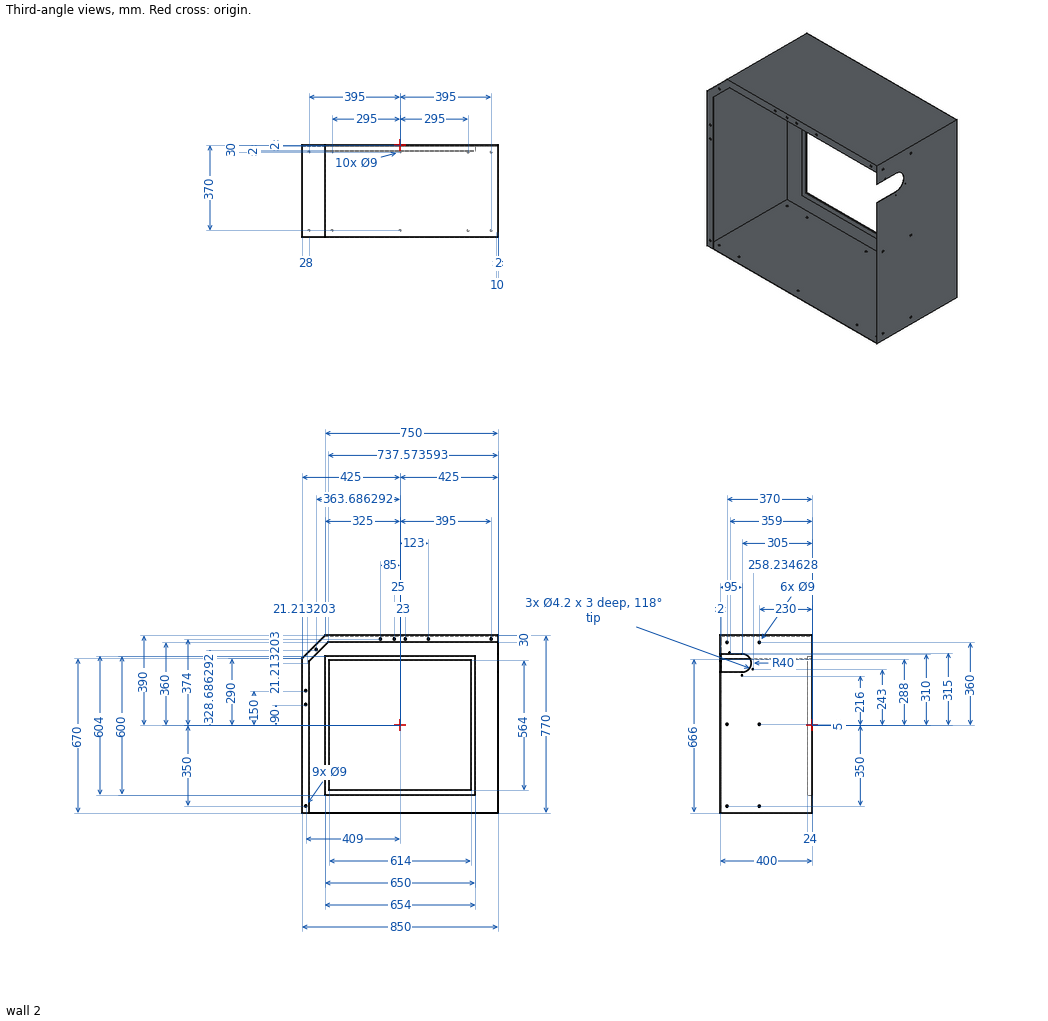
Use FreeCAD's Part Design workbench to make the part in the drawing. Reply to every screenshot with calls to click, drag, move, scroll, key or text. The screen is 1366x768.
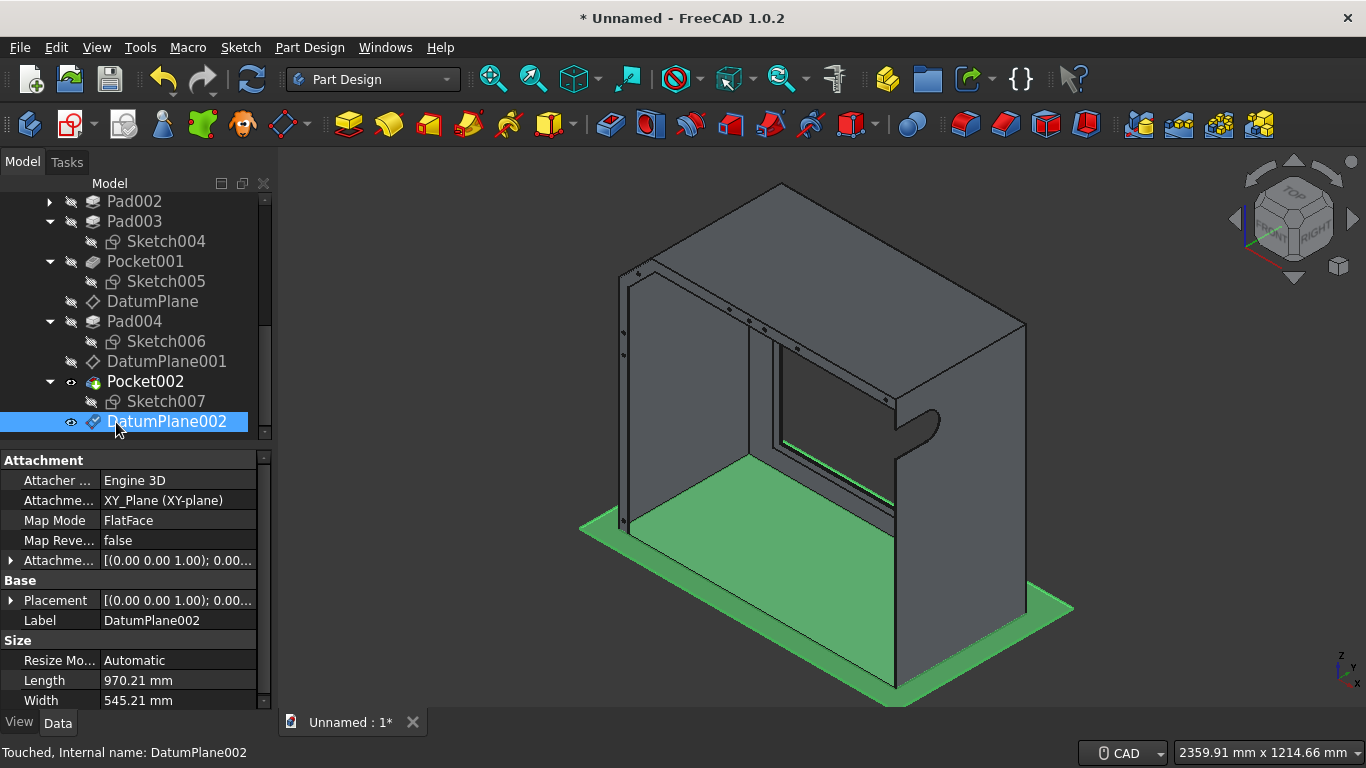
click(70, 124)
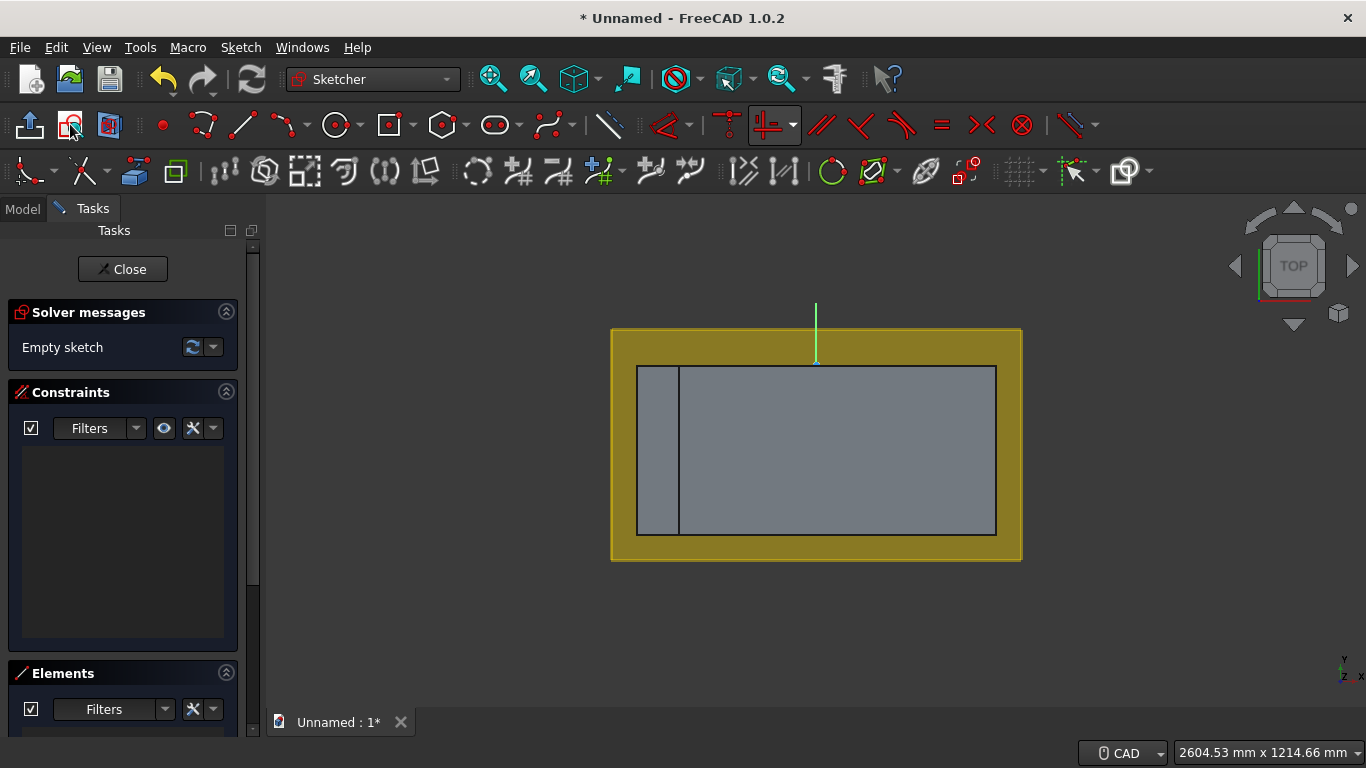
click(110, 126)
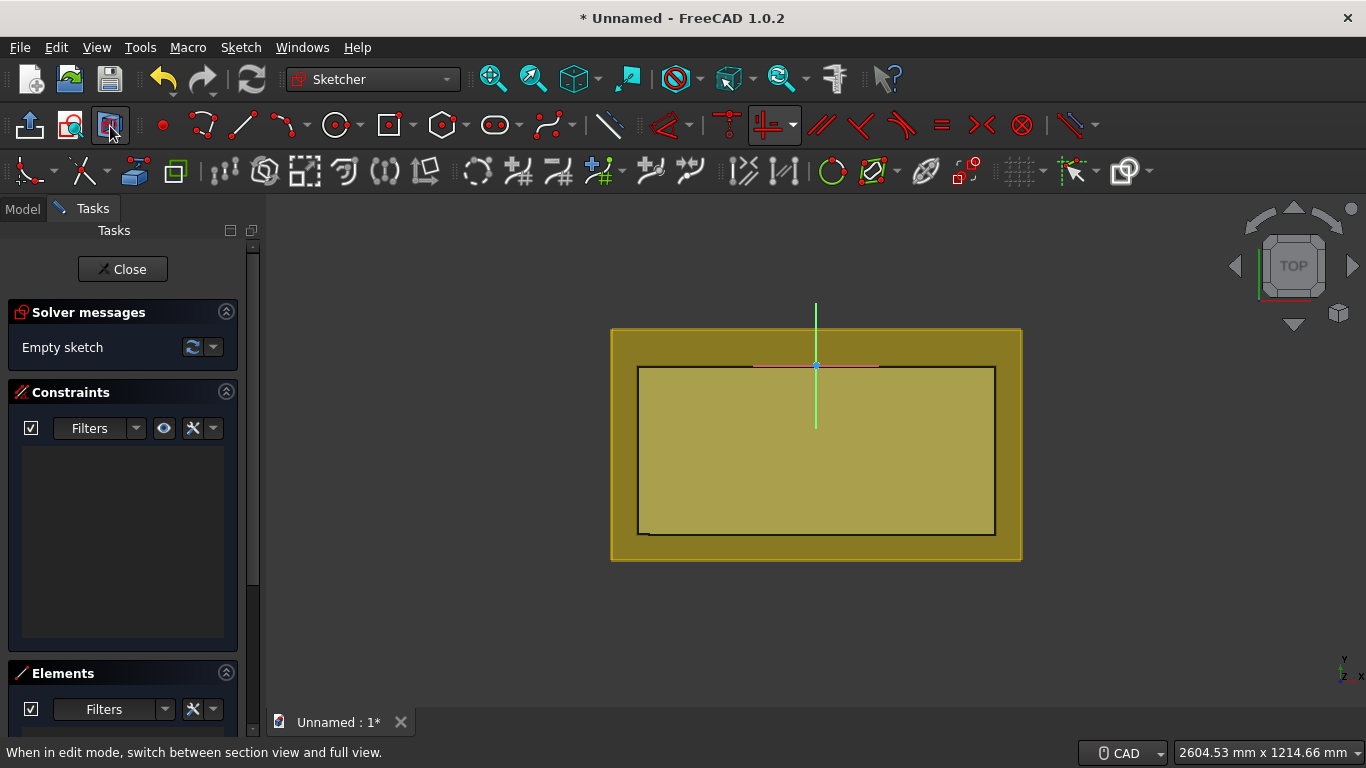
scroll(900, 438, up, 3)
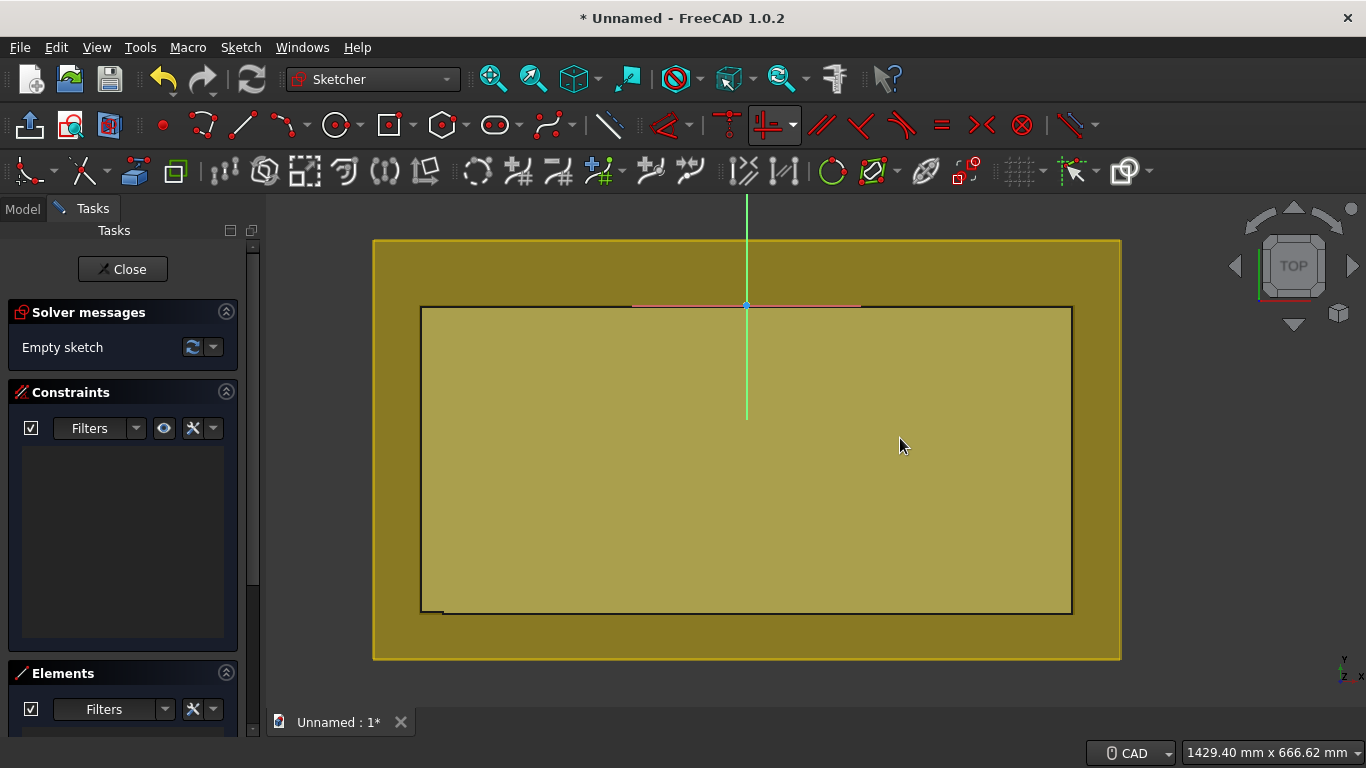
click(336, 126)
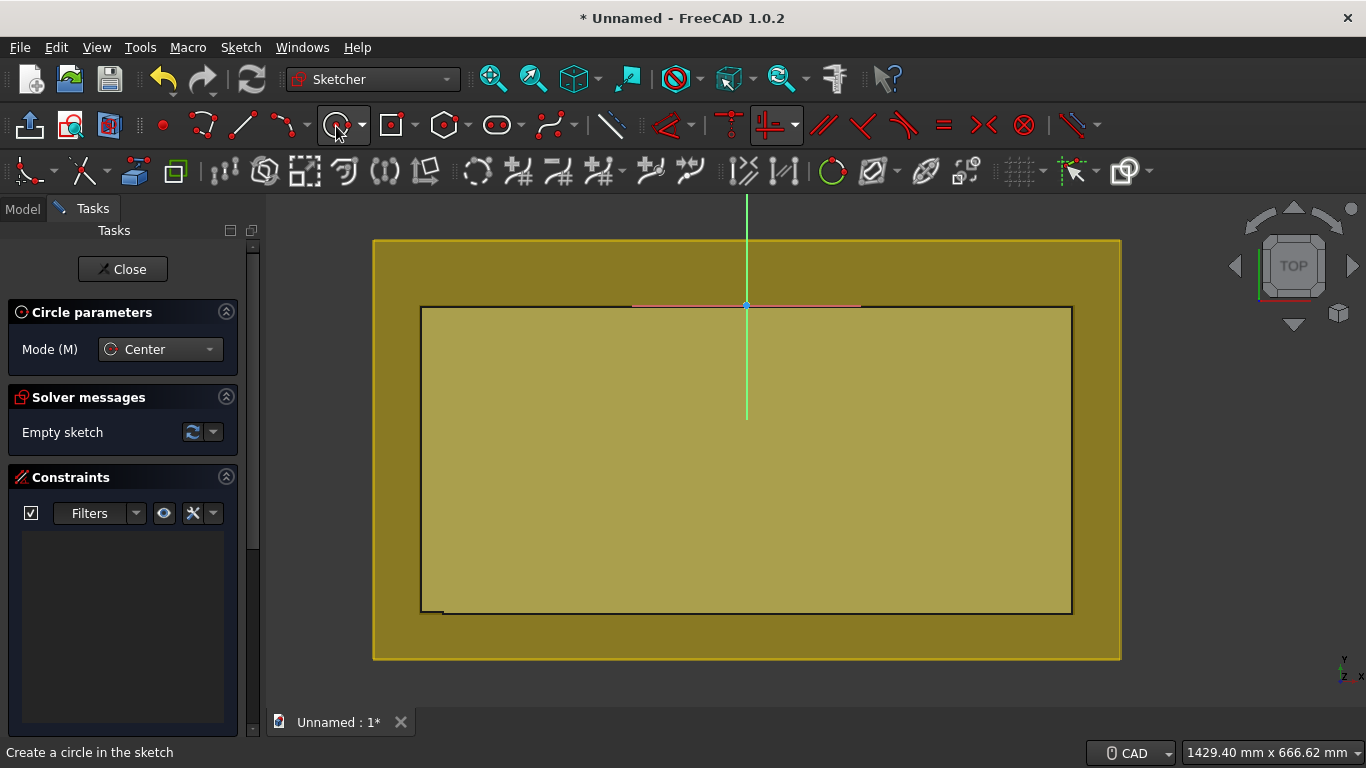
scroll(747, 329, up, 10)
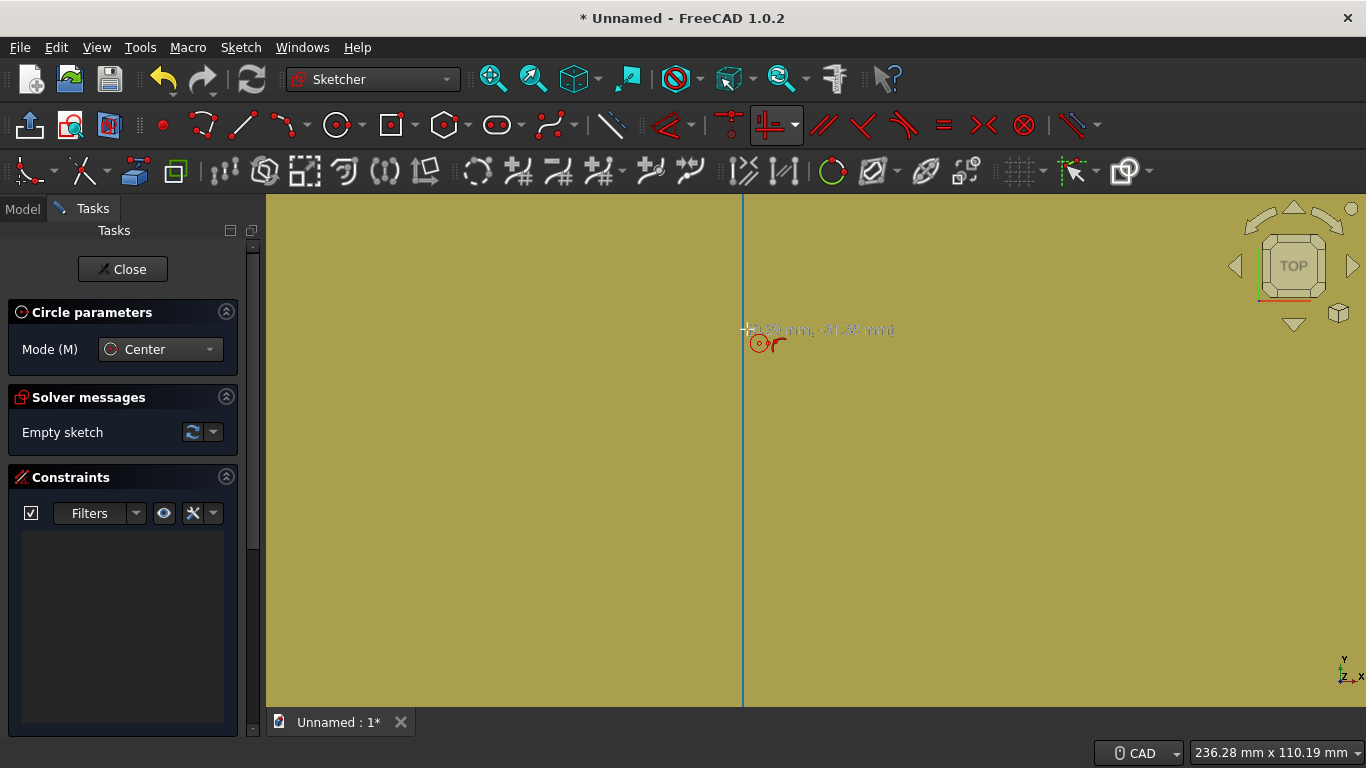
scroll(748, 330, down, 10)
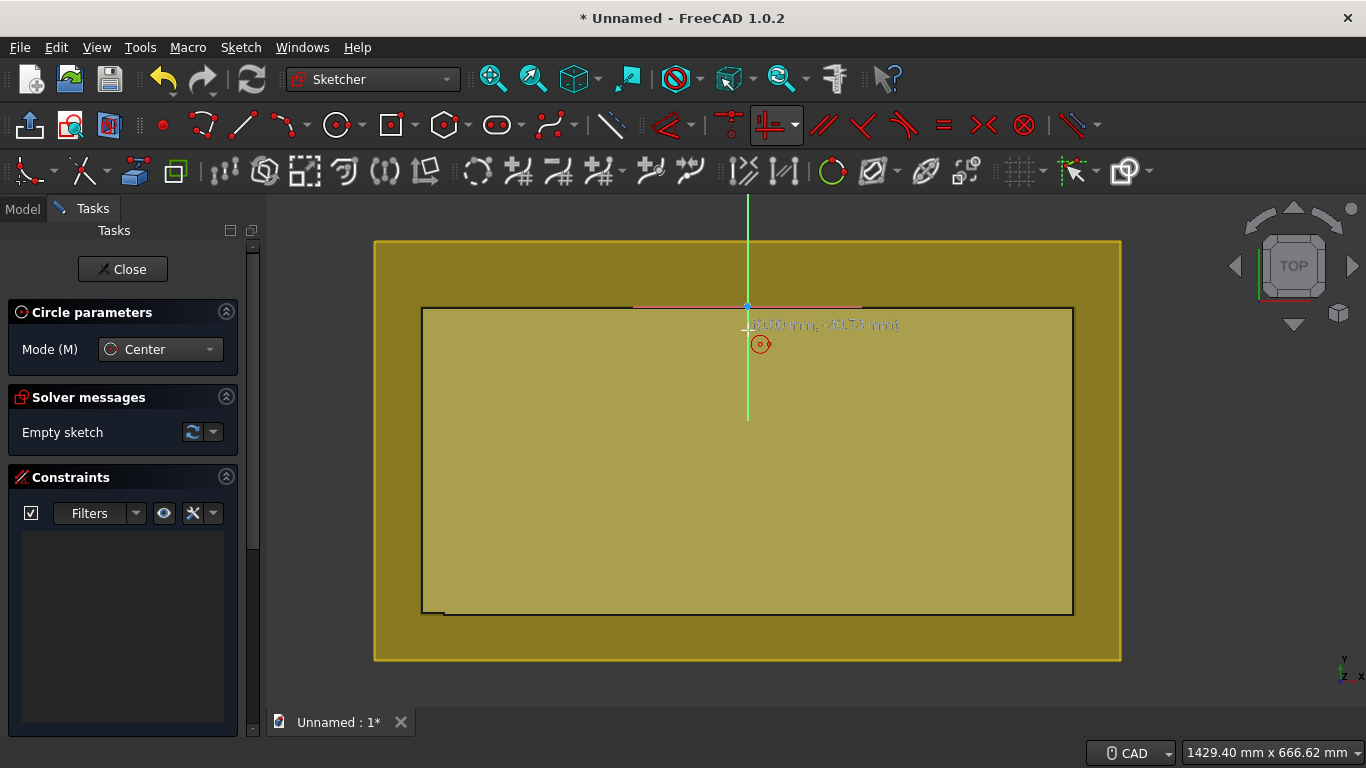
click(748, 330)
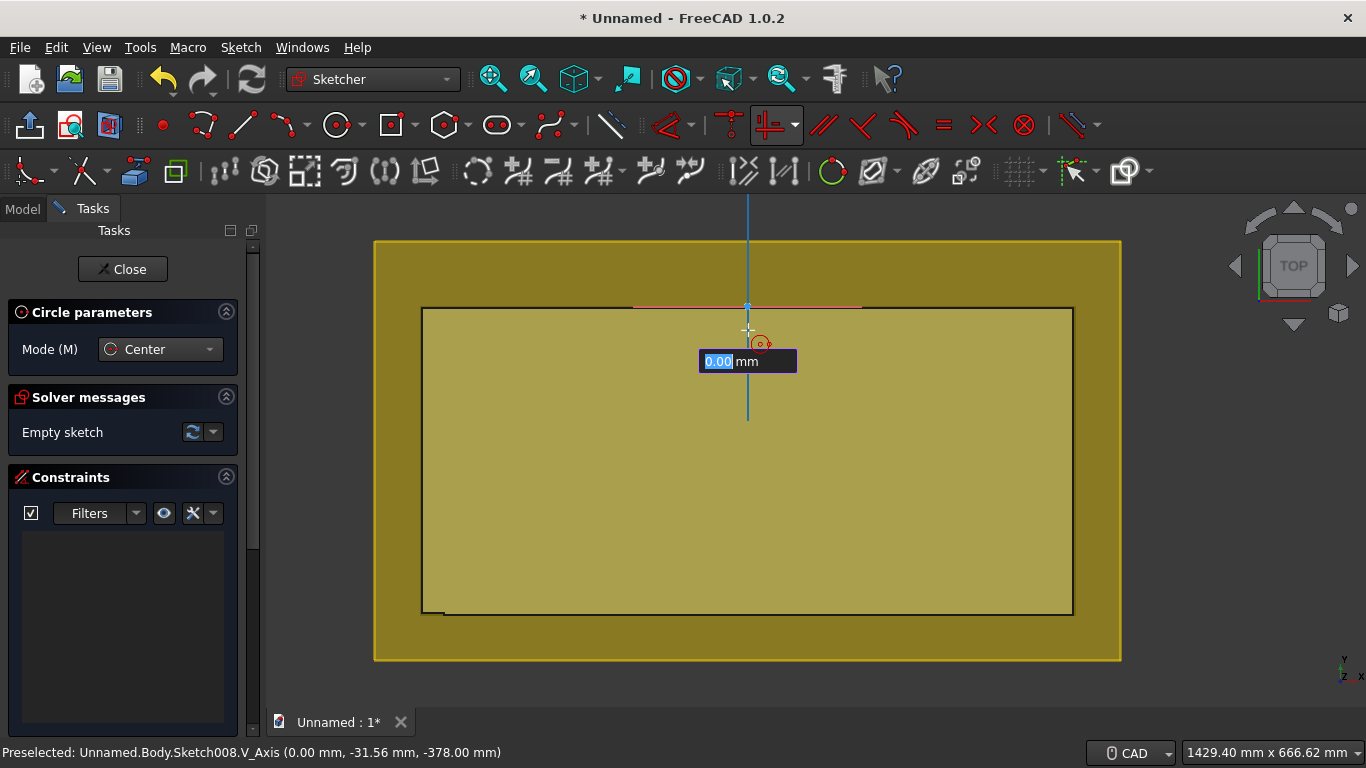
scroll(751, 329, up, 8)
move(749, 326)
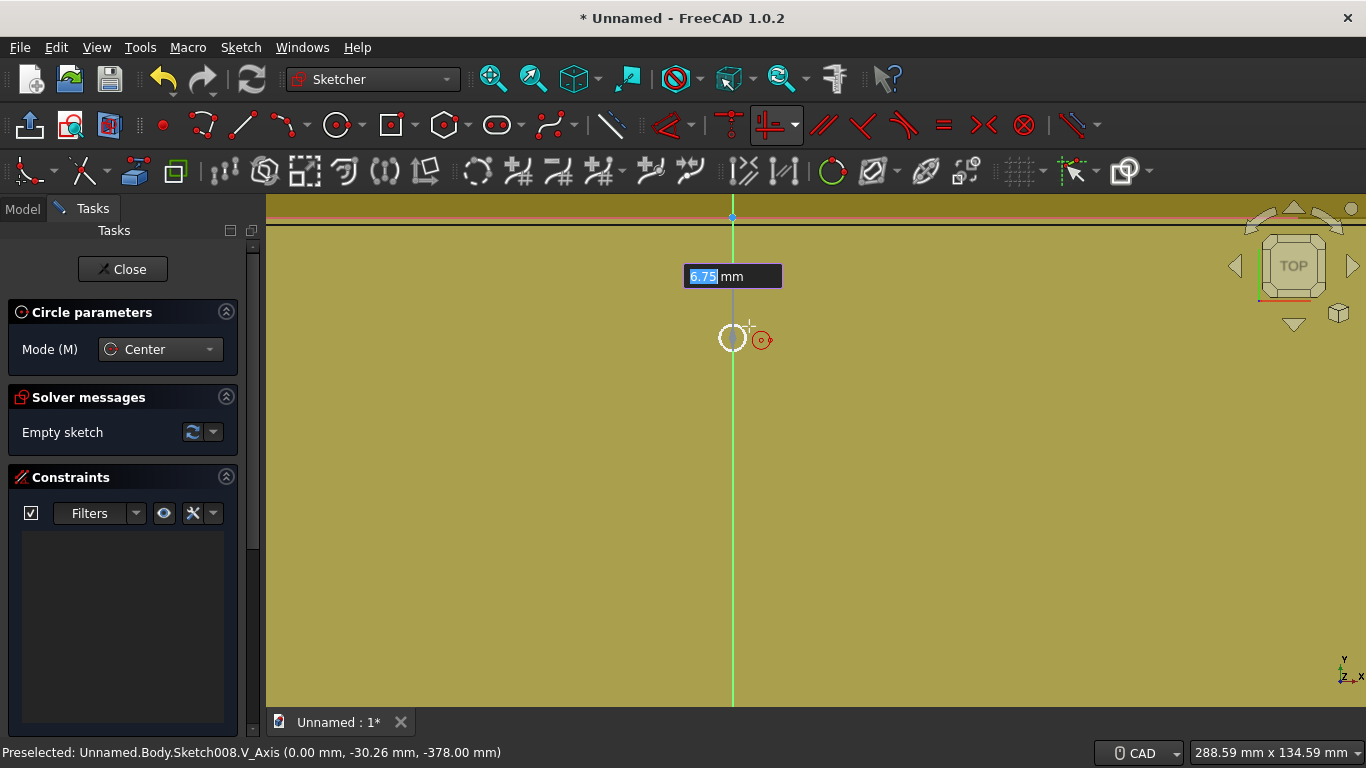
text(9)
key(Return)